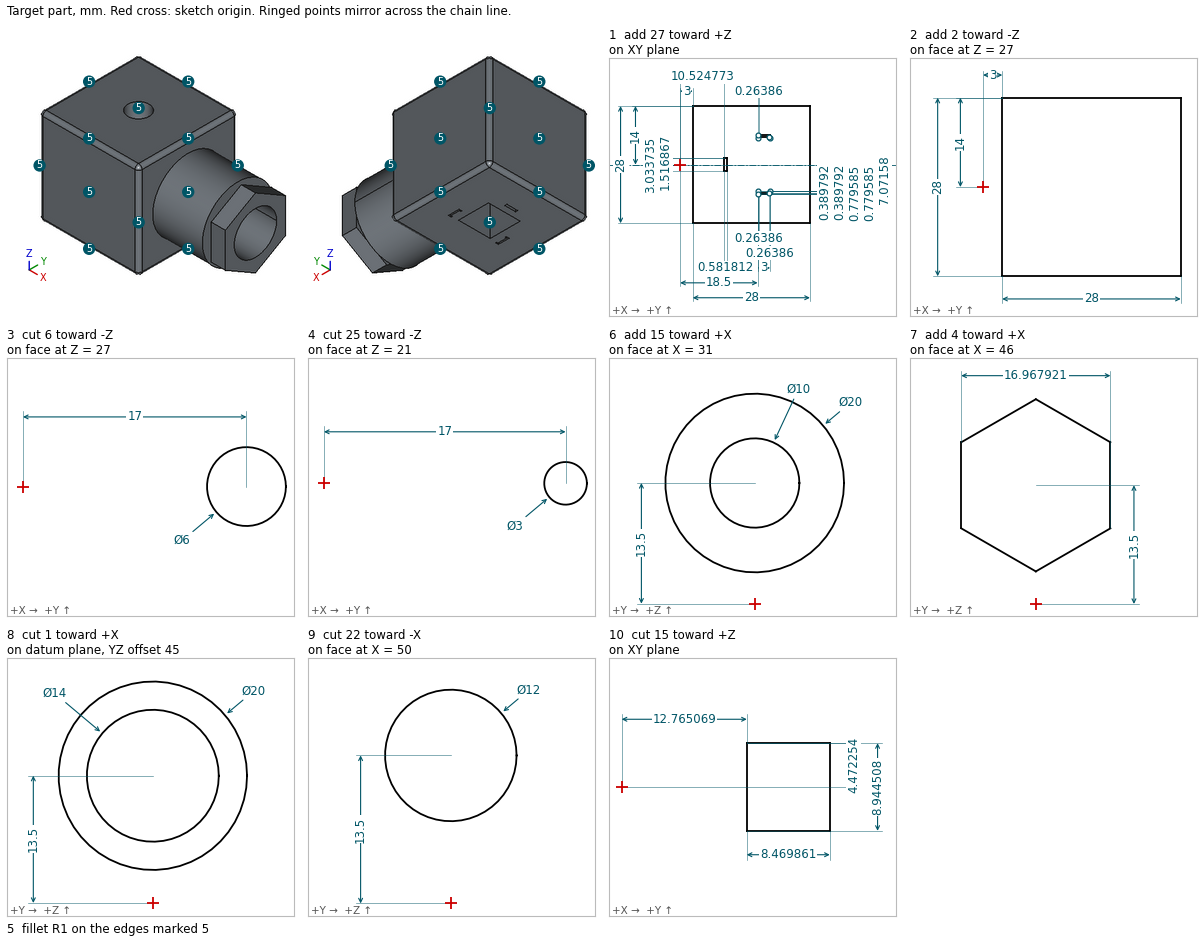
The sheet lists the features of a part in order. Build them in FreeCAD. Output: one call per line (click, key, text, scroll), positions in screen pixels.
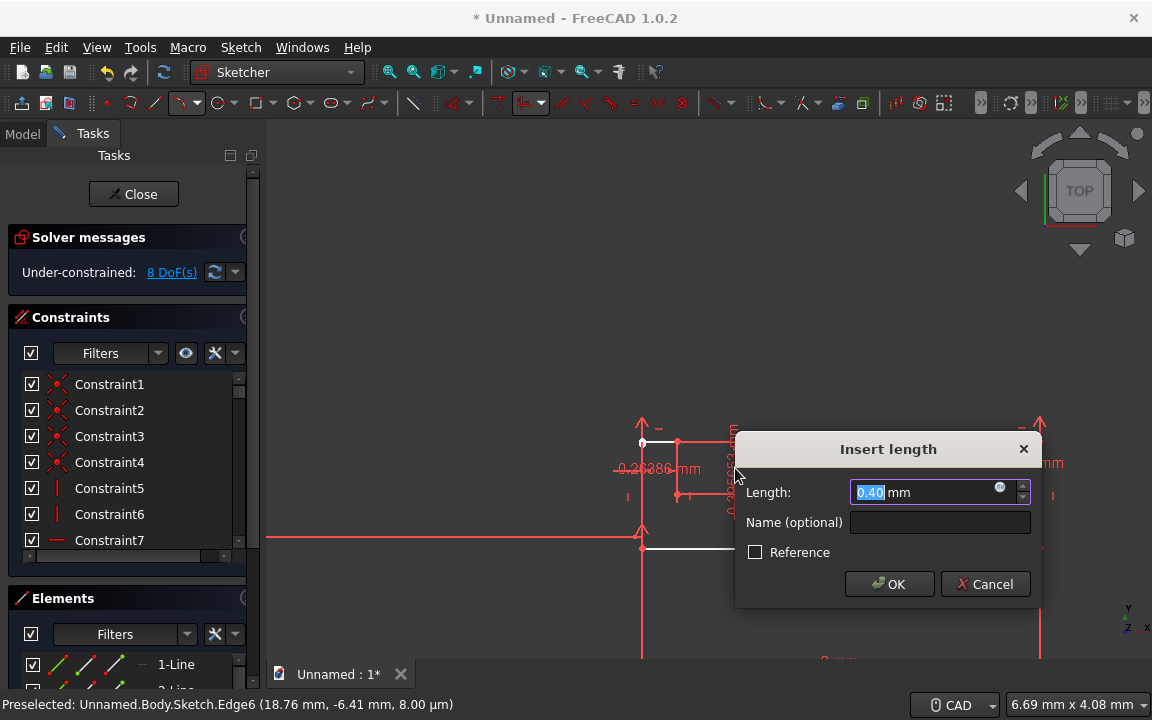
text(0.389792)
key(Return)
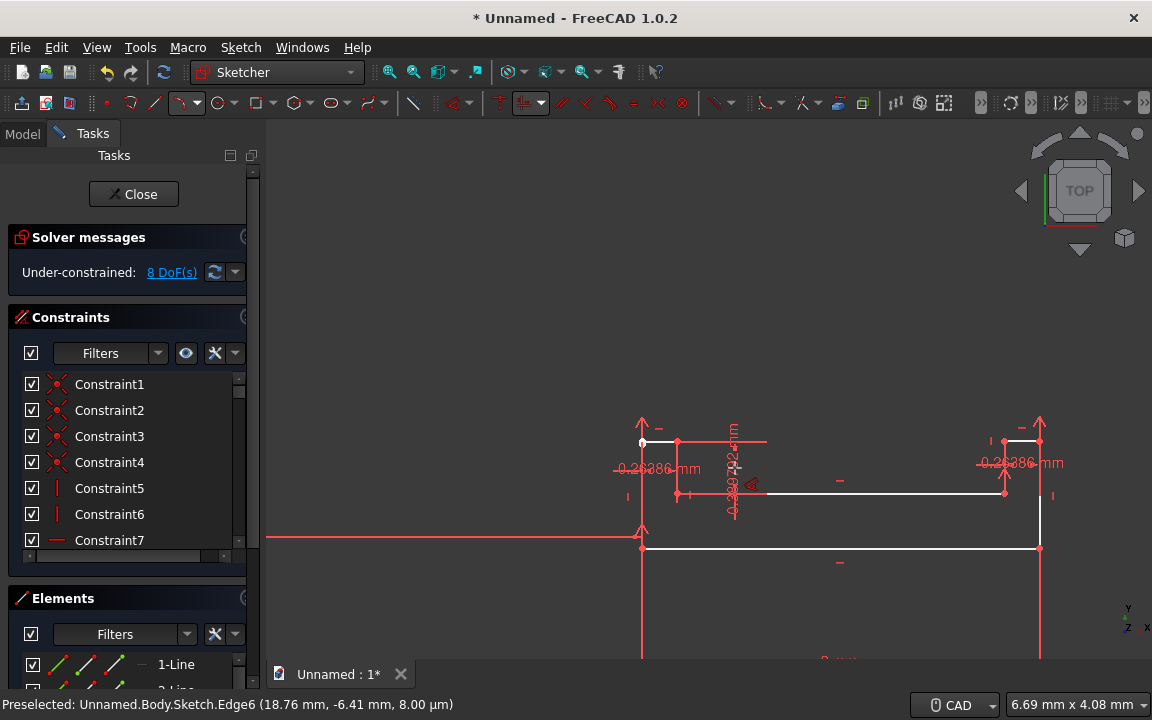
scroll(680, 467, down, 12)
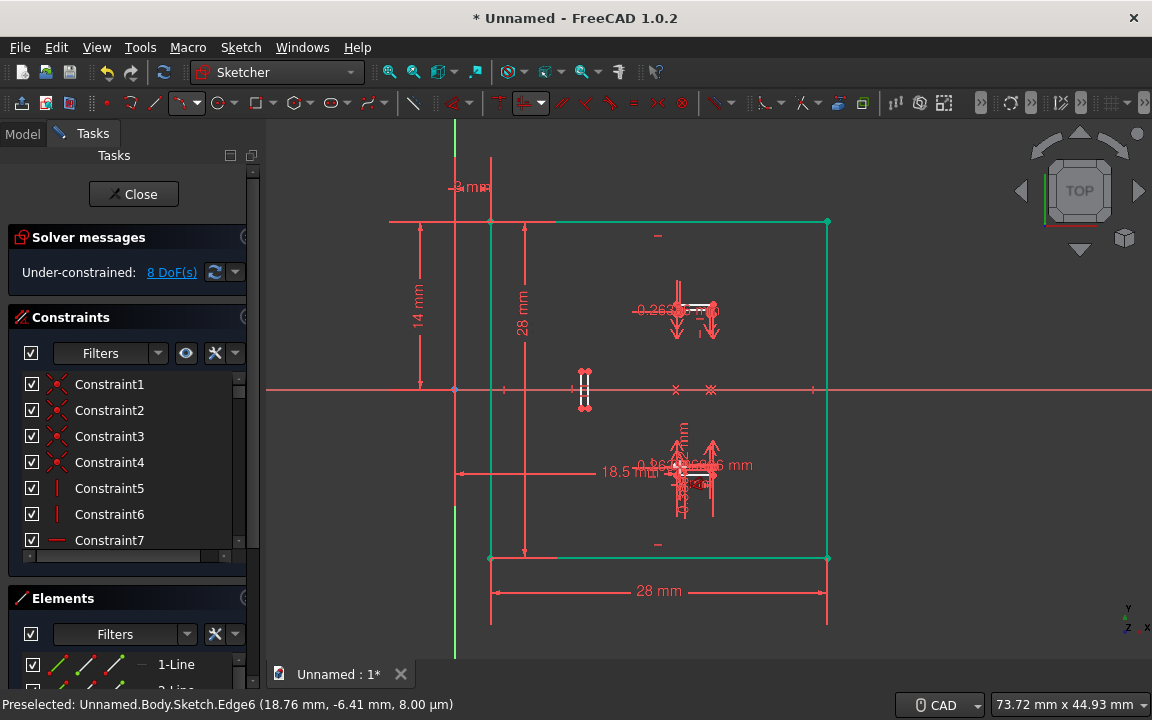
scroll(710, 469, up, 12)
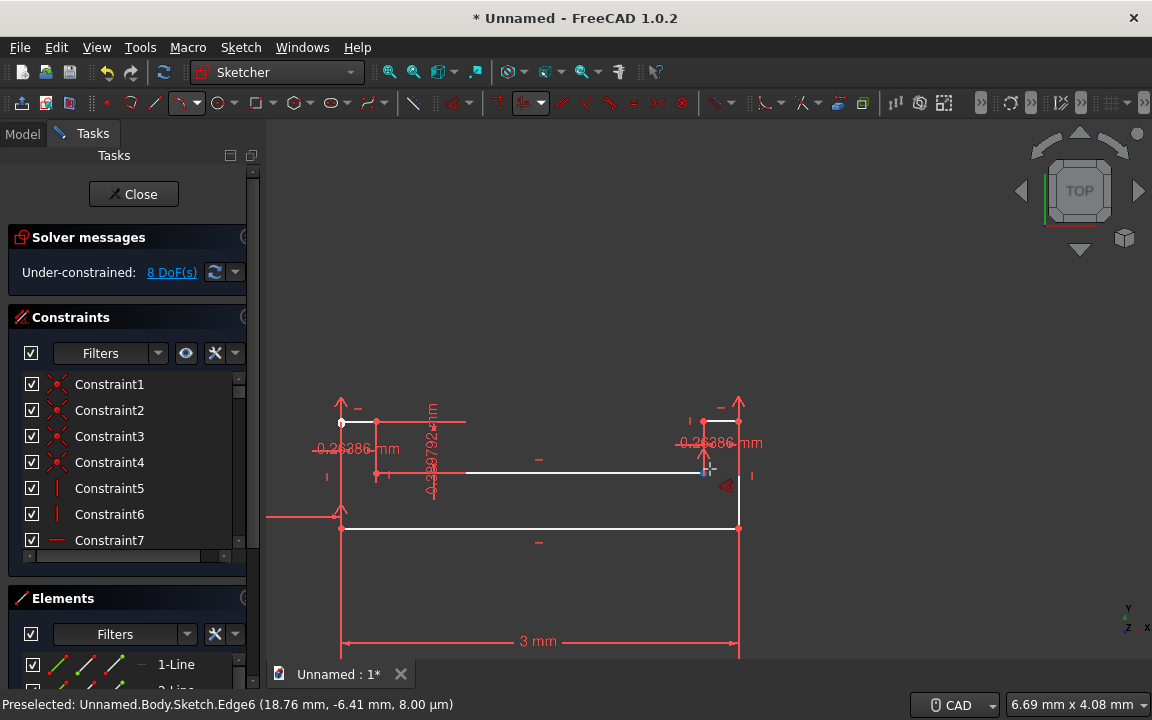
click(704, 458)
click(762, 466)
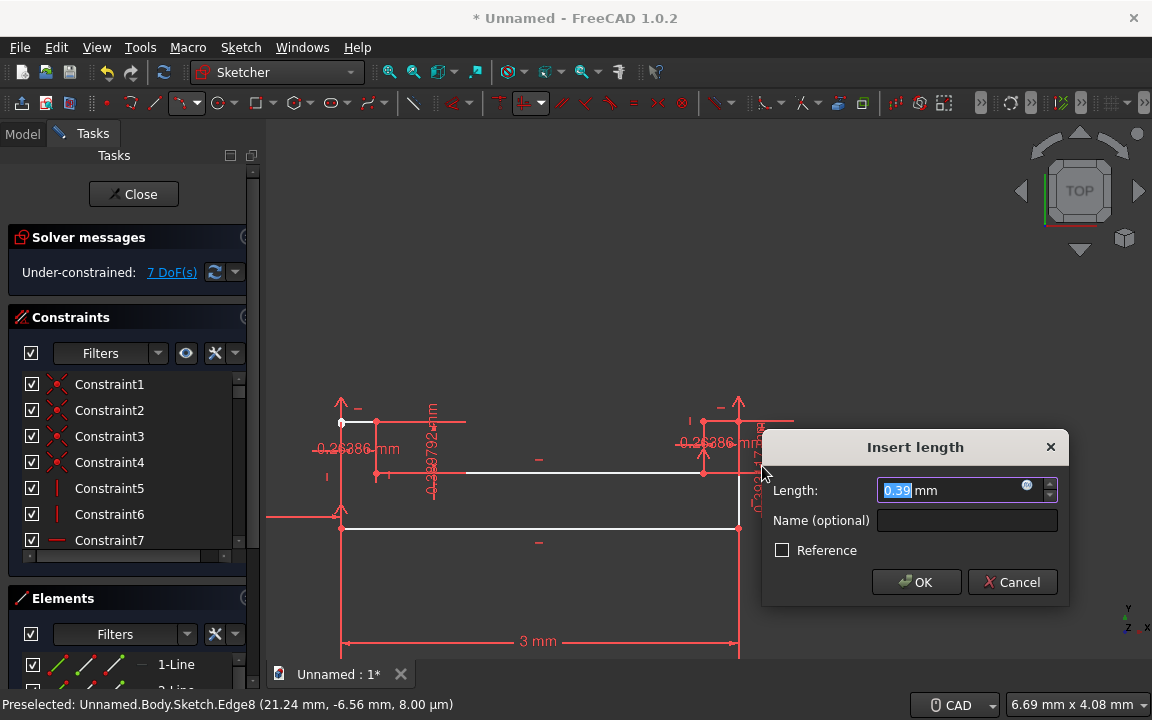
text(0.389792)
key(Return)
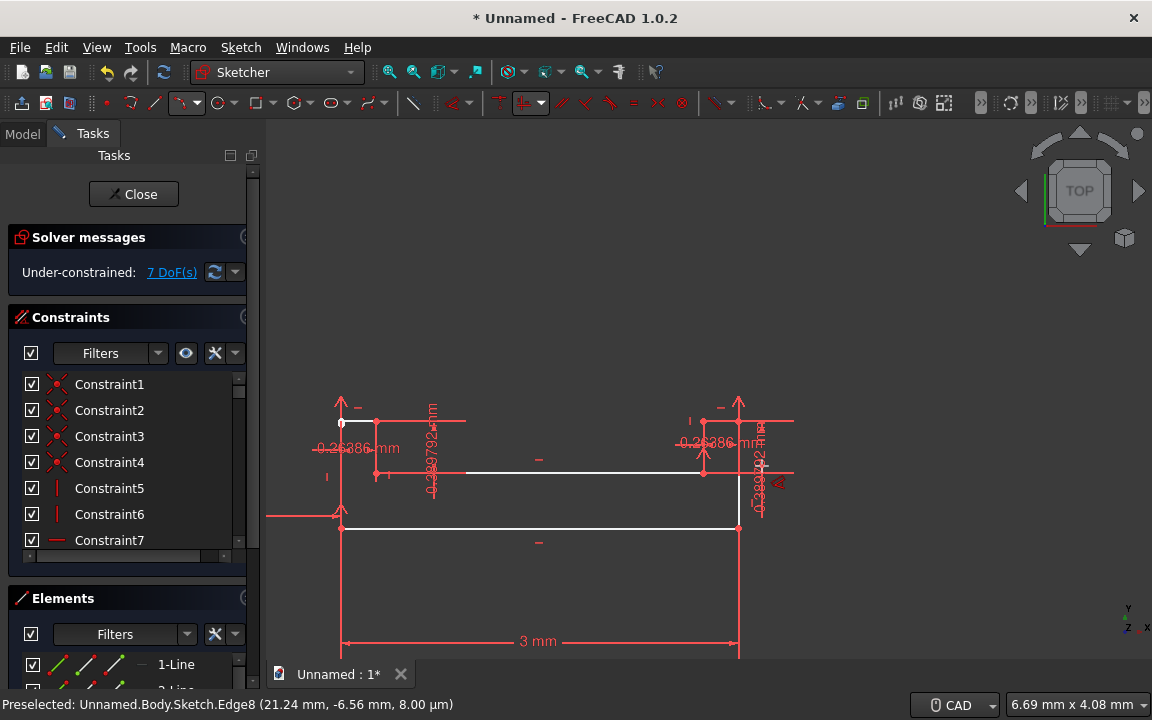
click(739, 454)
click(773, 500)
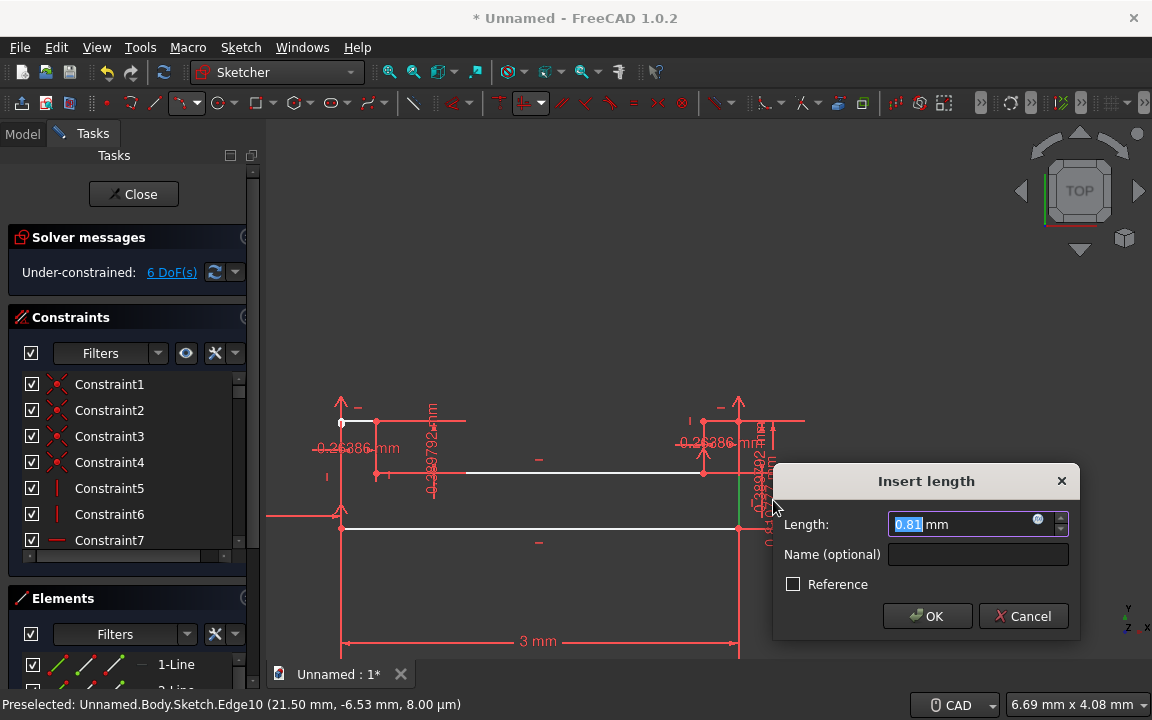
text(0.779585)
key(Return)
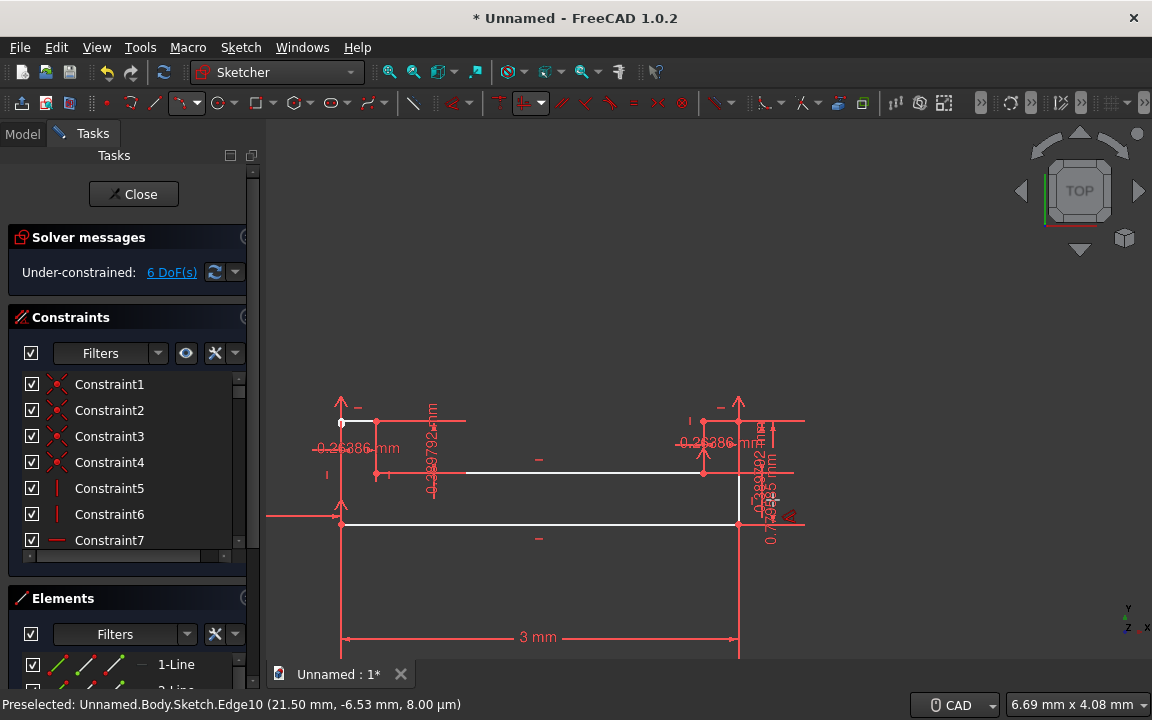
click(341, 495)
click(375, 498)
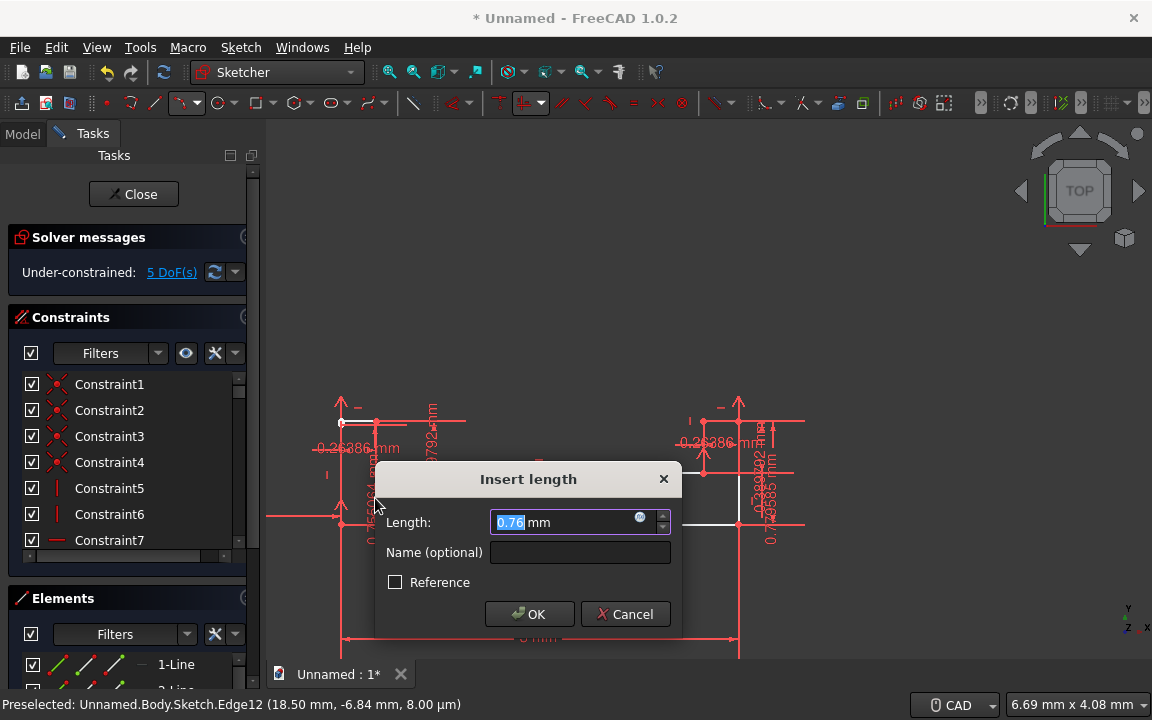
text(0.779585)
key(Return)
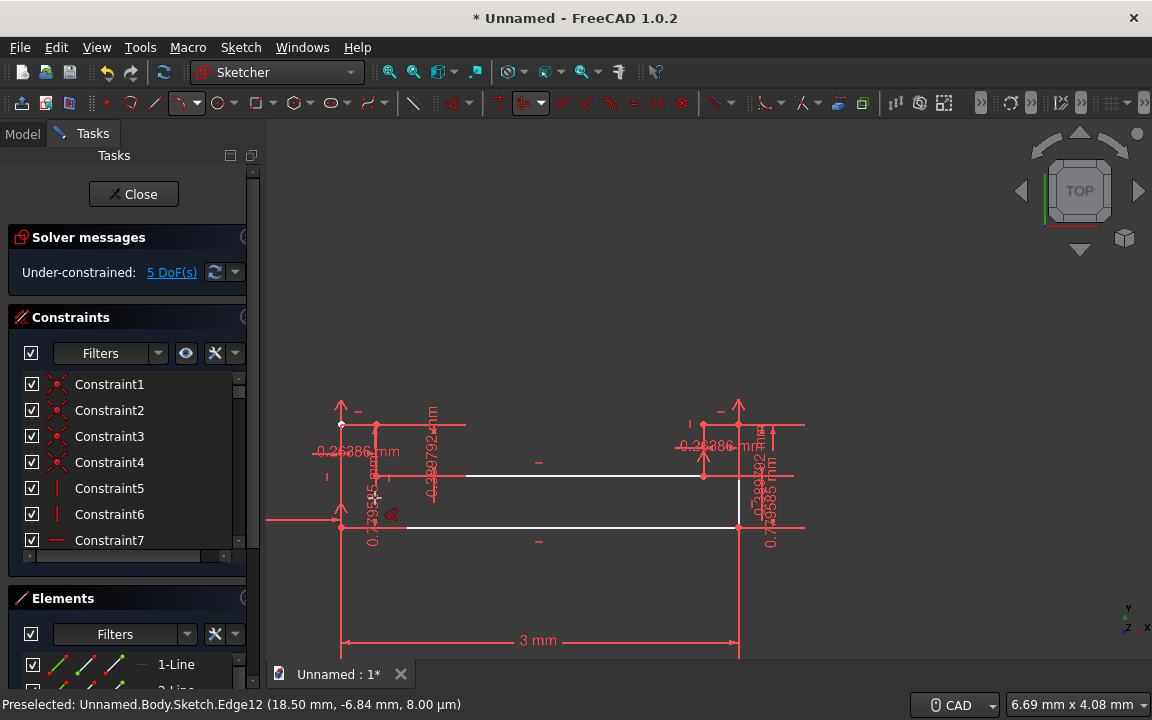
scroll(710, 469, down, 12)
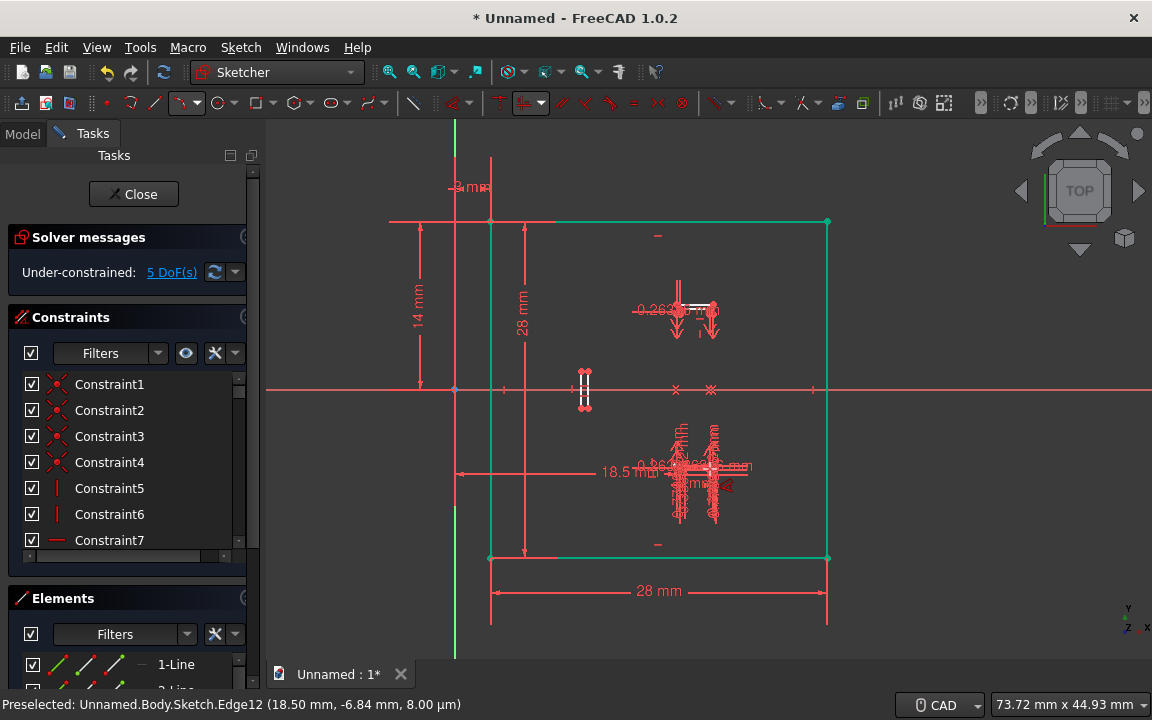
scroll(581, 383, up, 4)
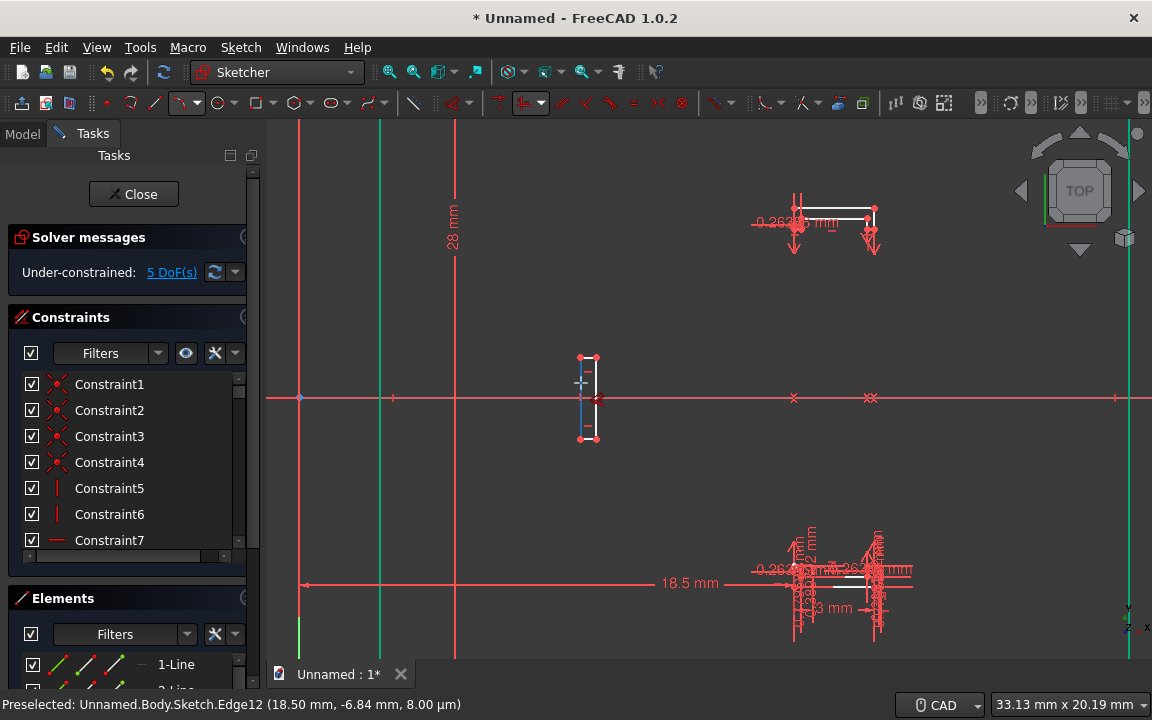
click(581, 382)
click(547, 380)